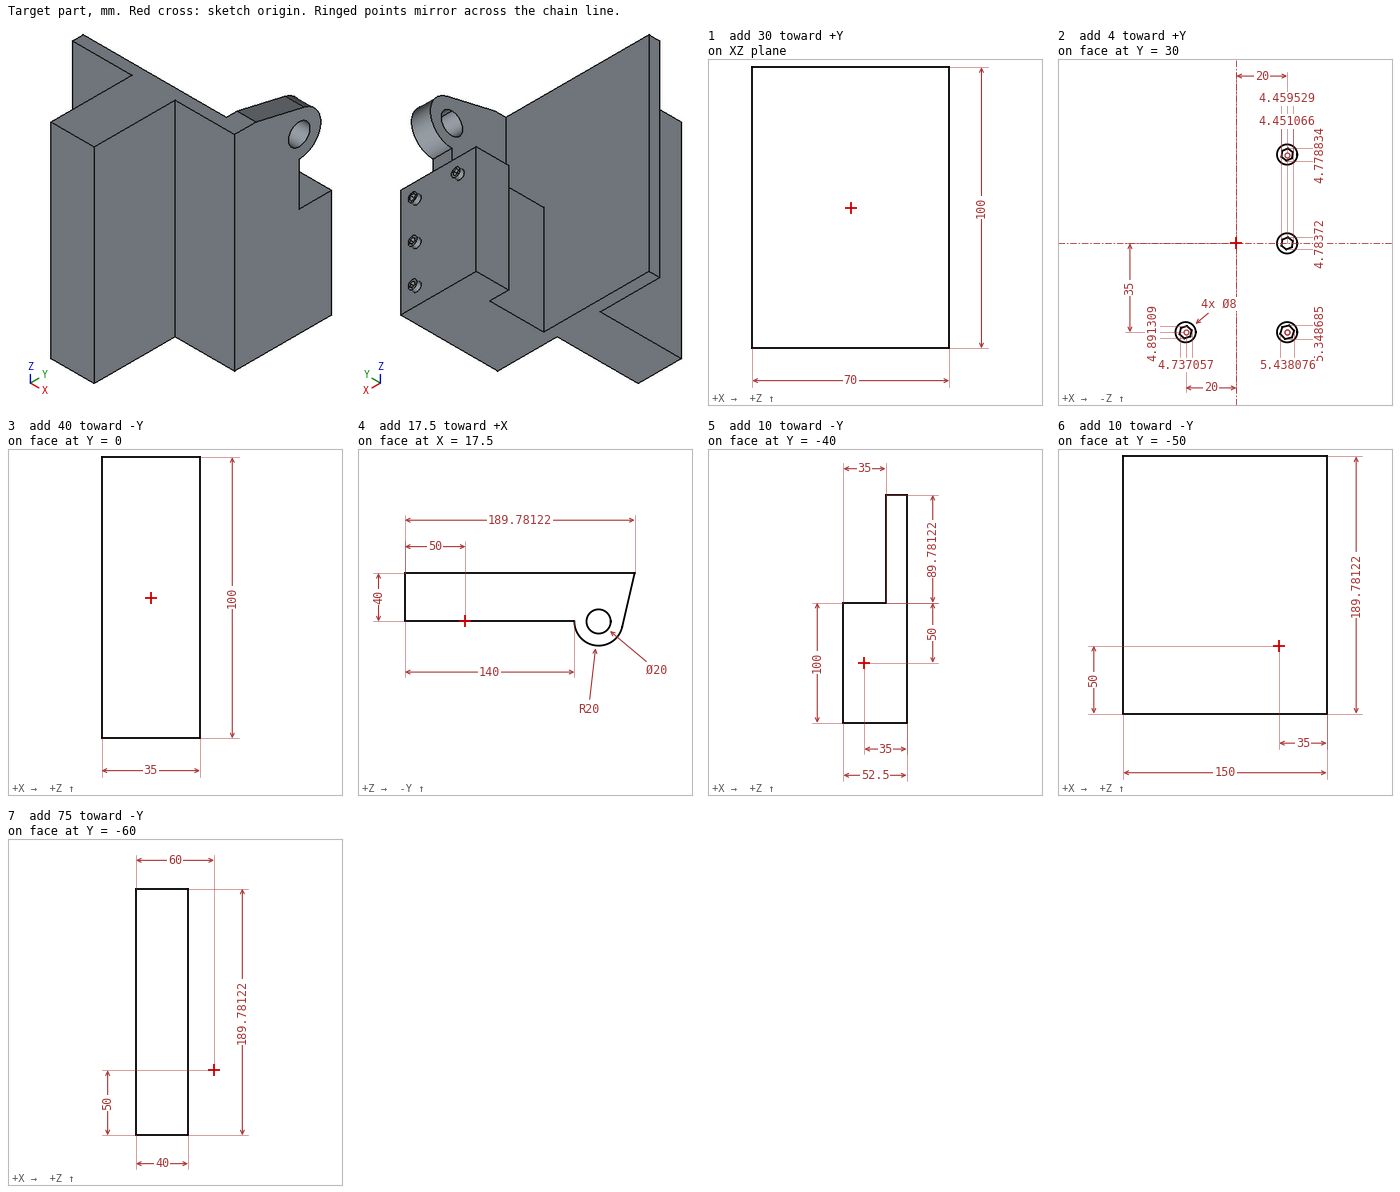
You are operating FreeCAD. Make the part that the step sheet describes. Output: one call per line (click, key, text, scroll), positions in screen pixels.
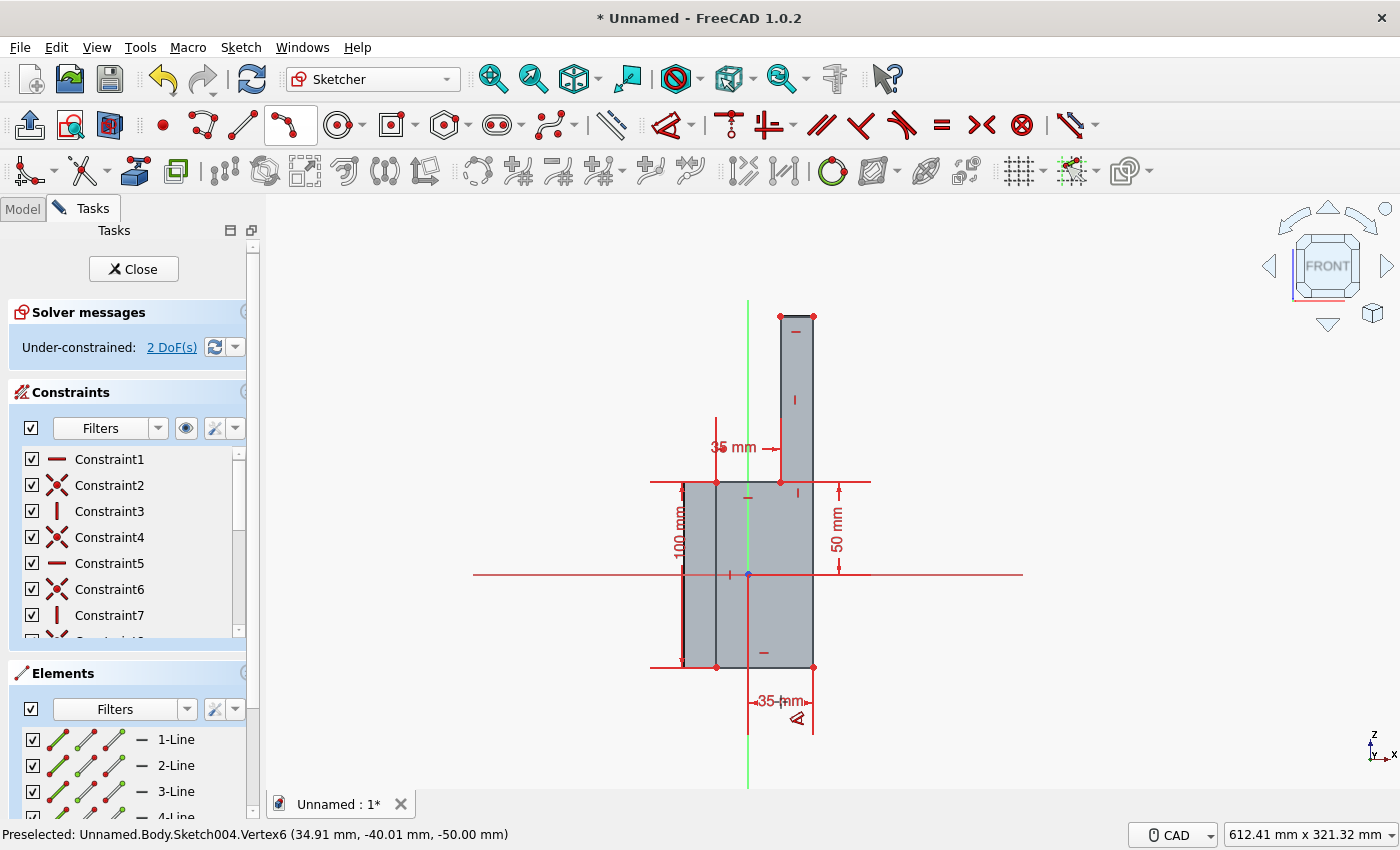
click(745, 668)
click(765, 634)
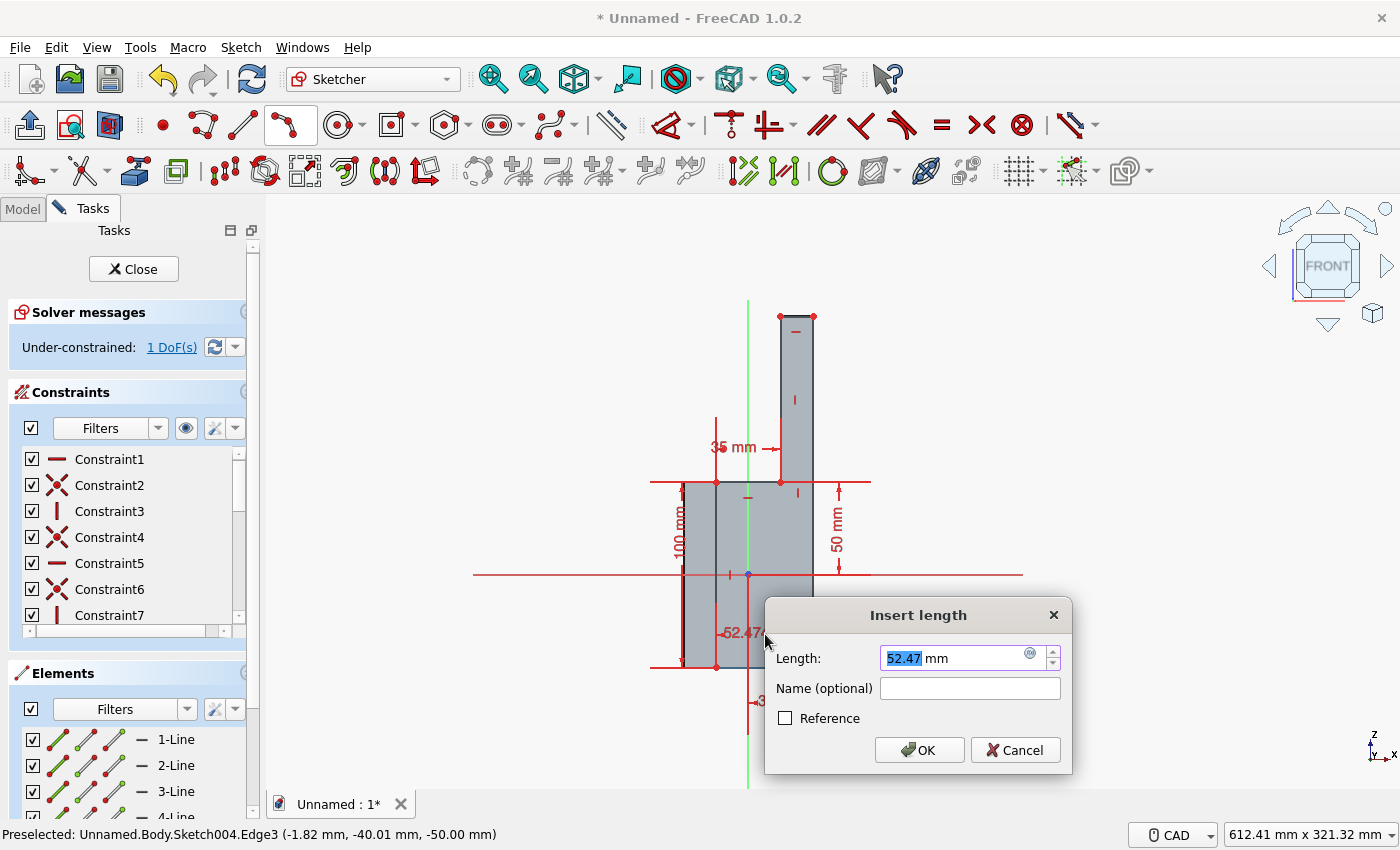
text(52.5)
key(Return)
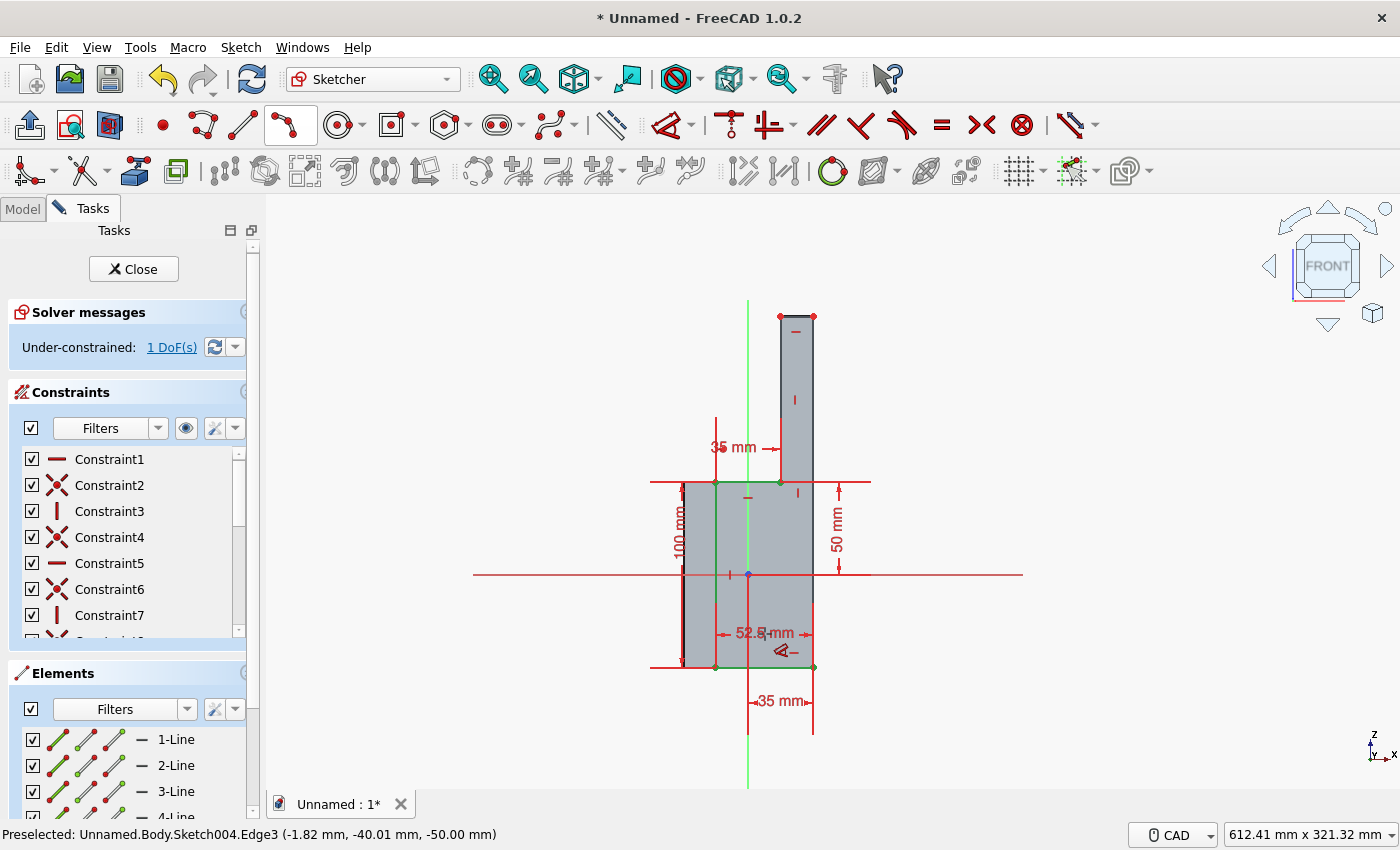
click(781, 367)
click(839, 400)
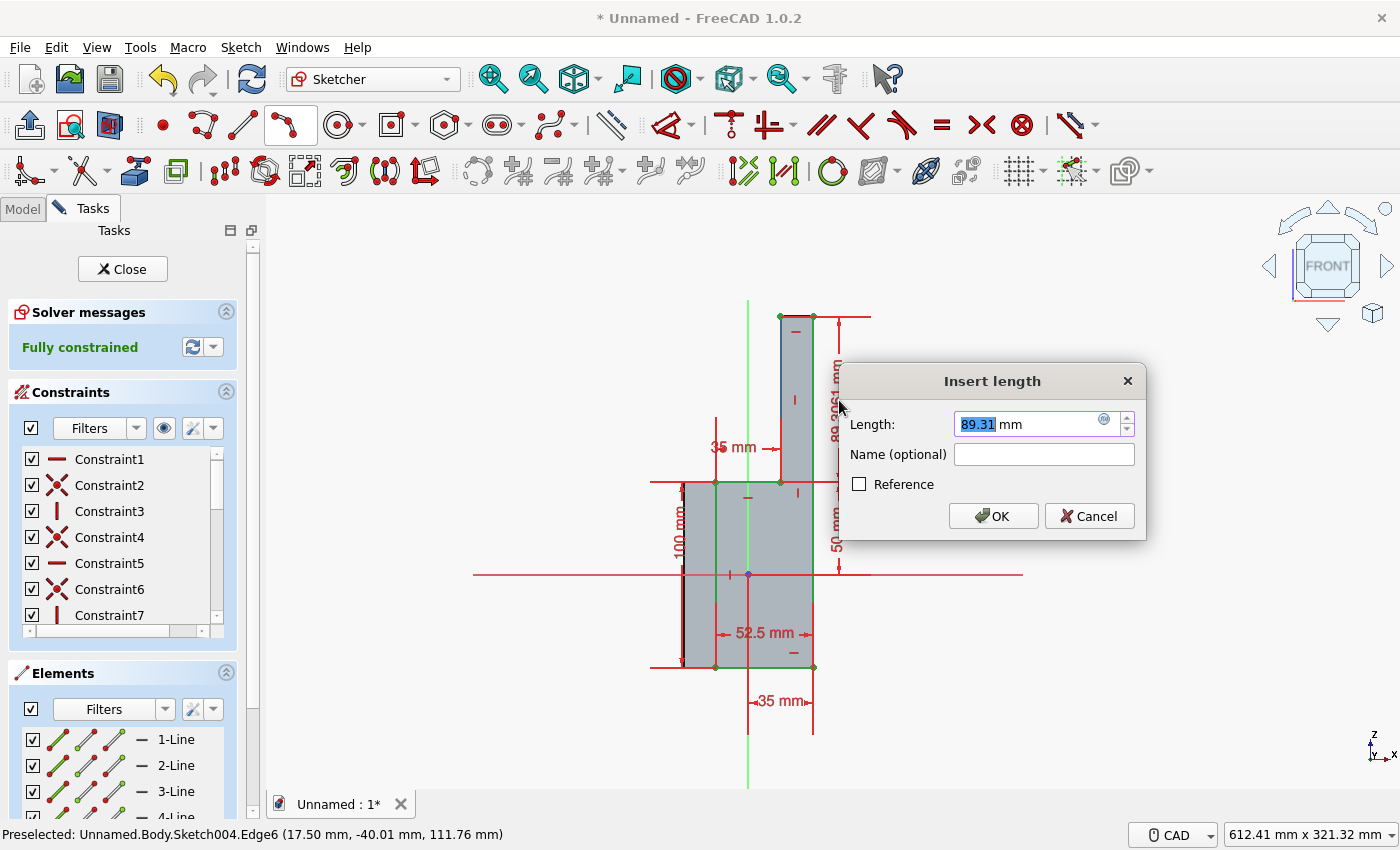
text(89.78122)
key(Return)
key(Escape)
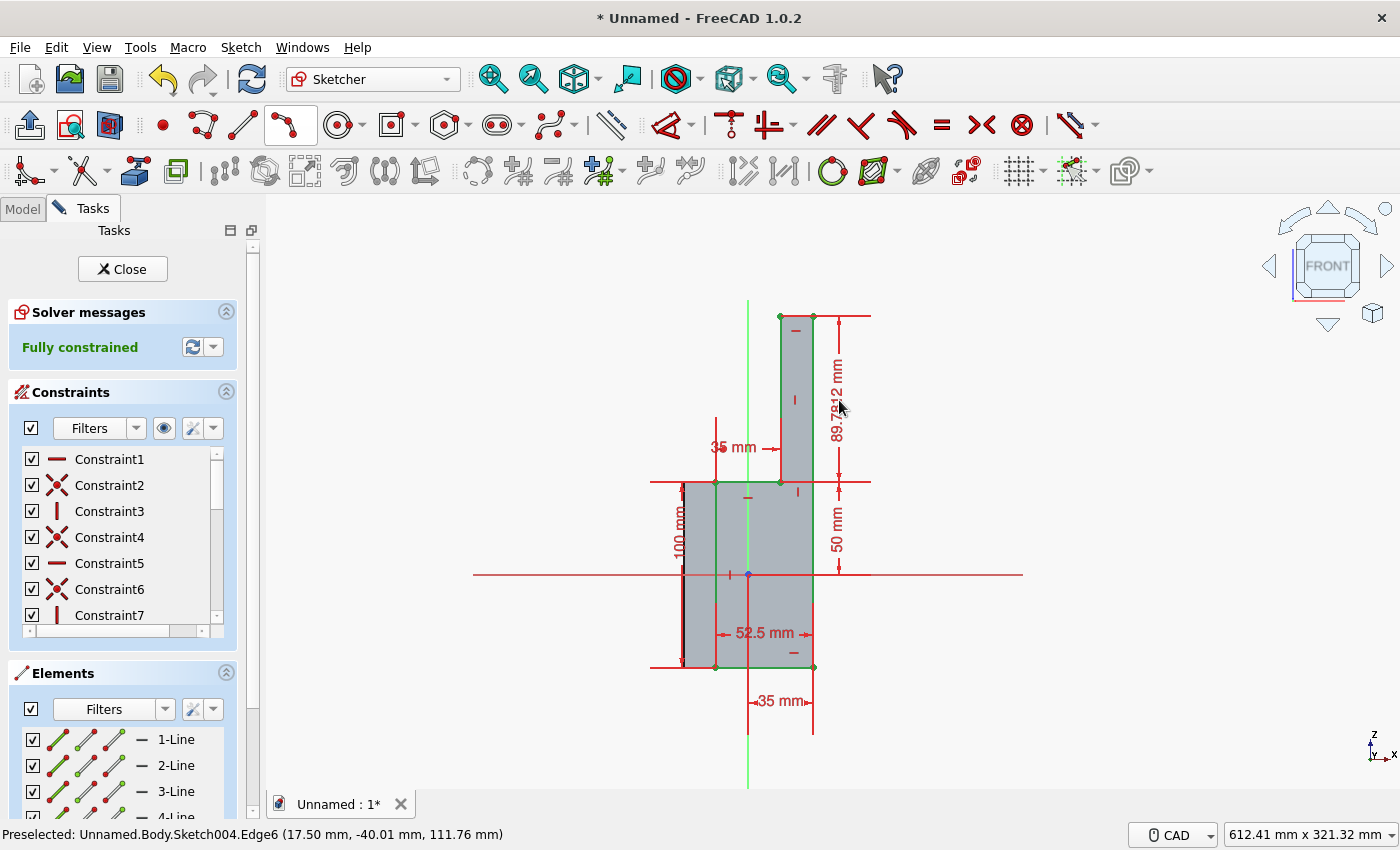
click(123, 269)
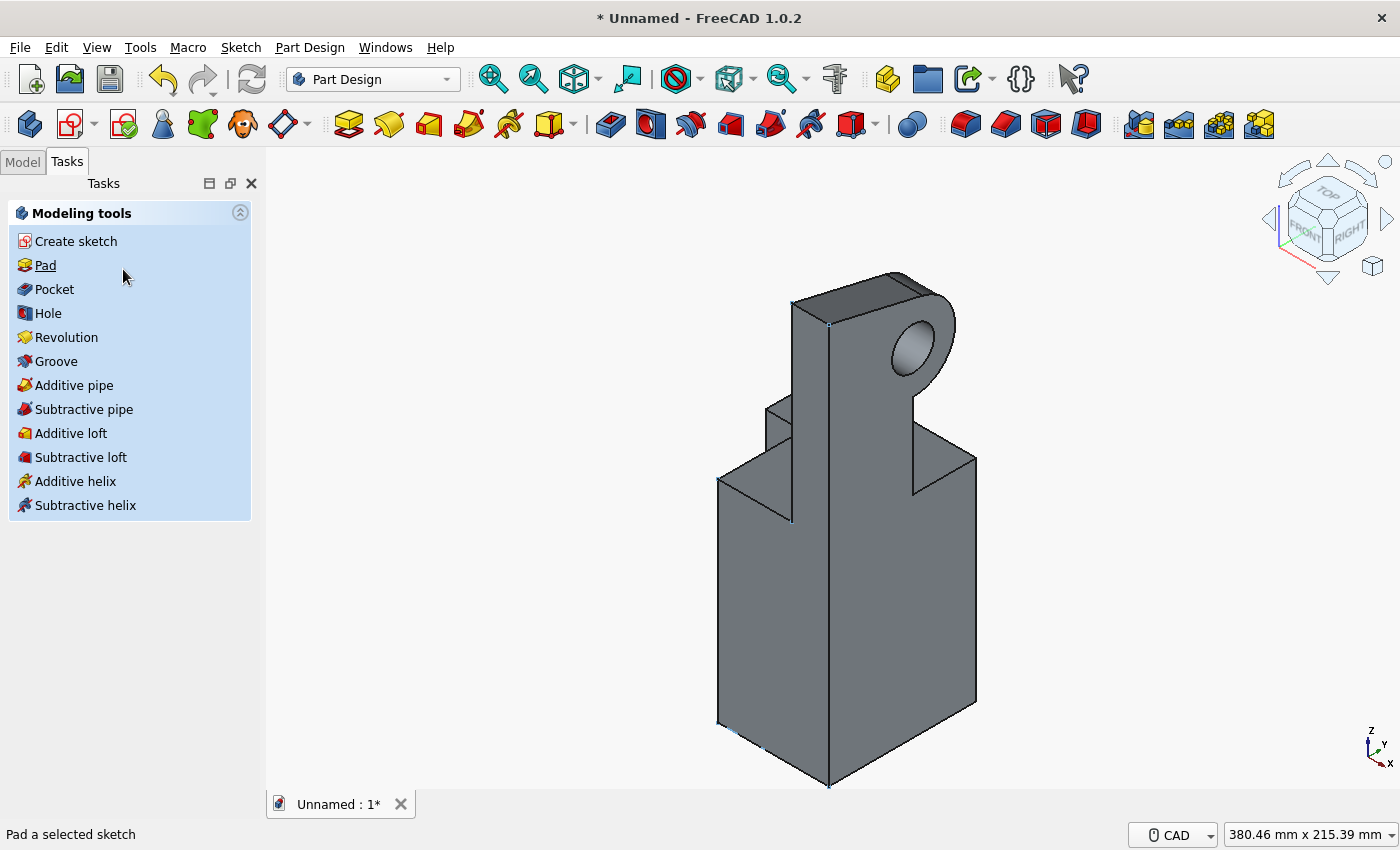
click(350, 124)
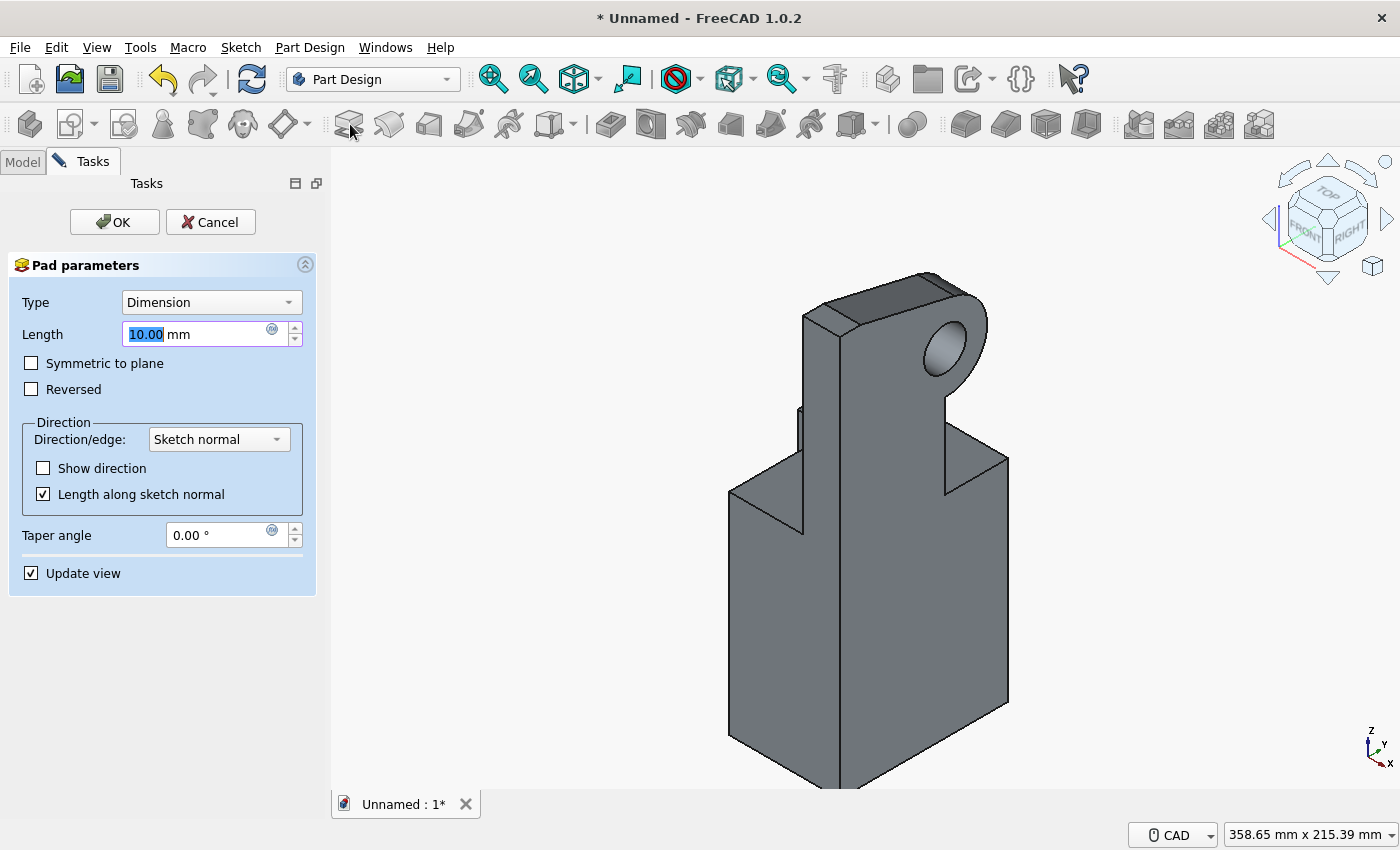
text(10)
key(Tab)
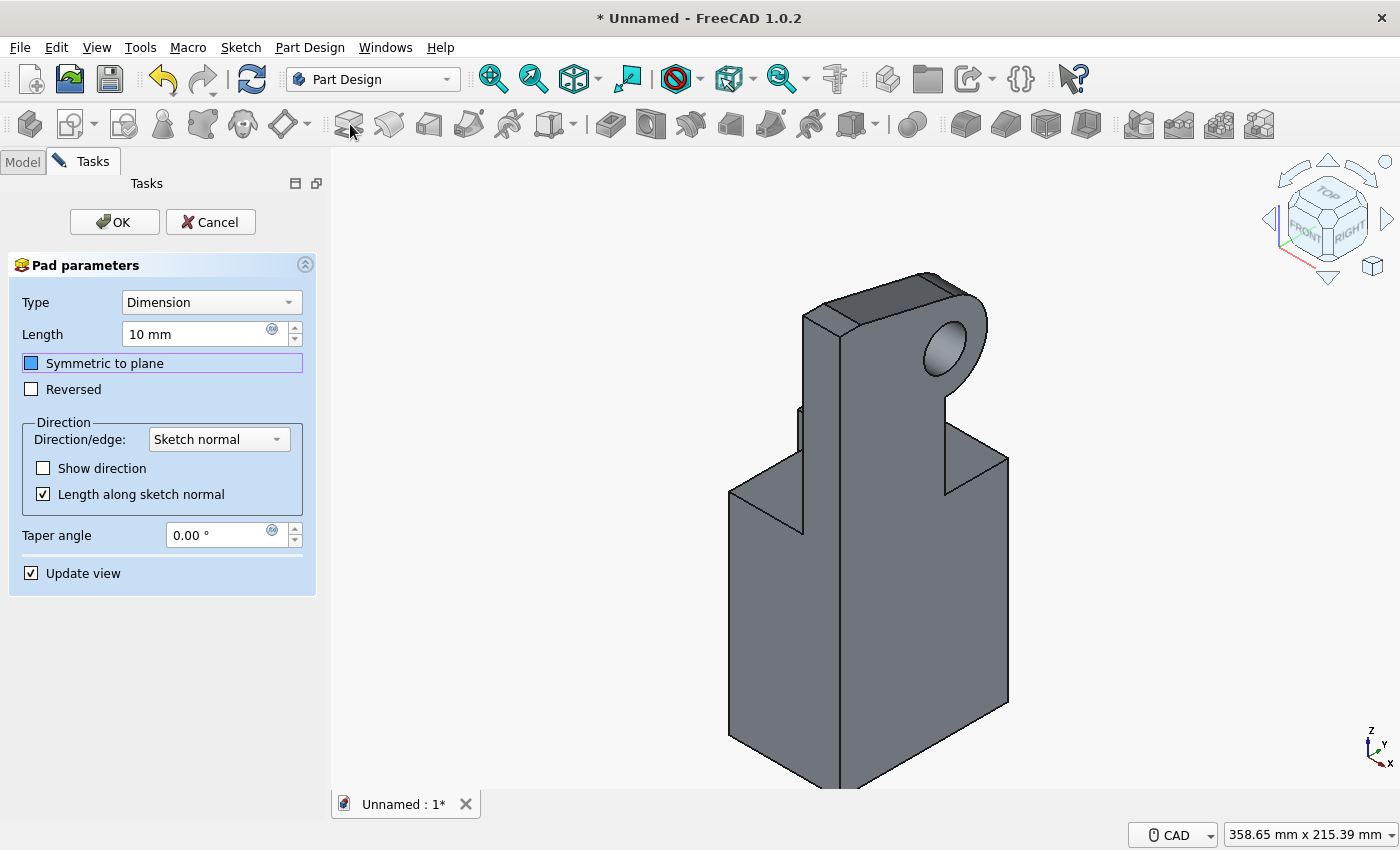
click(115, 222)